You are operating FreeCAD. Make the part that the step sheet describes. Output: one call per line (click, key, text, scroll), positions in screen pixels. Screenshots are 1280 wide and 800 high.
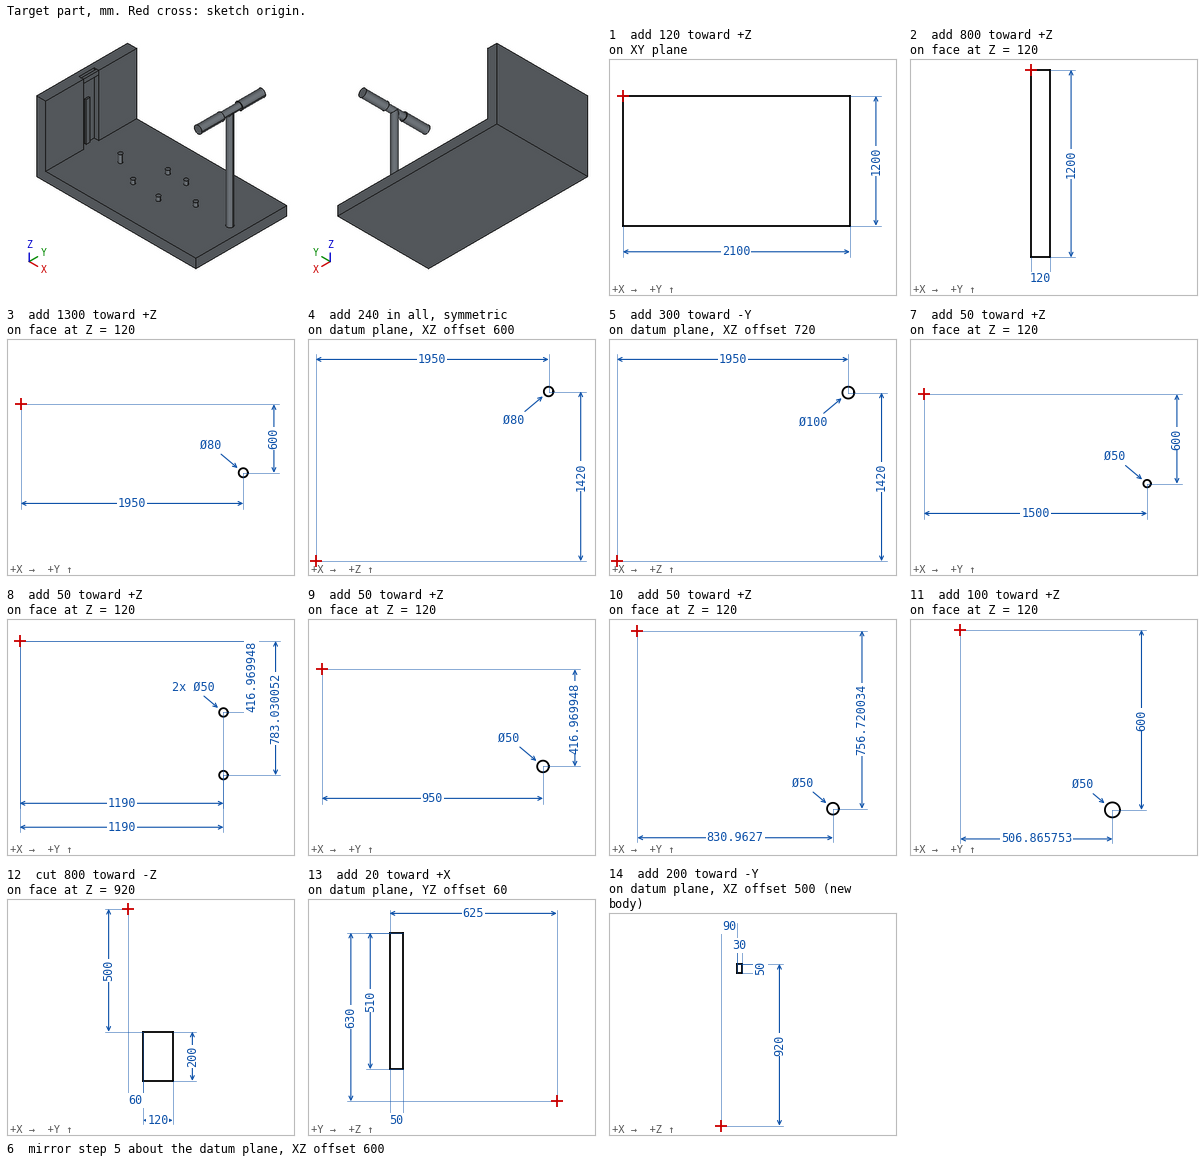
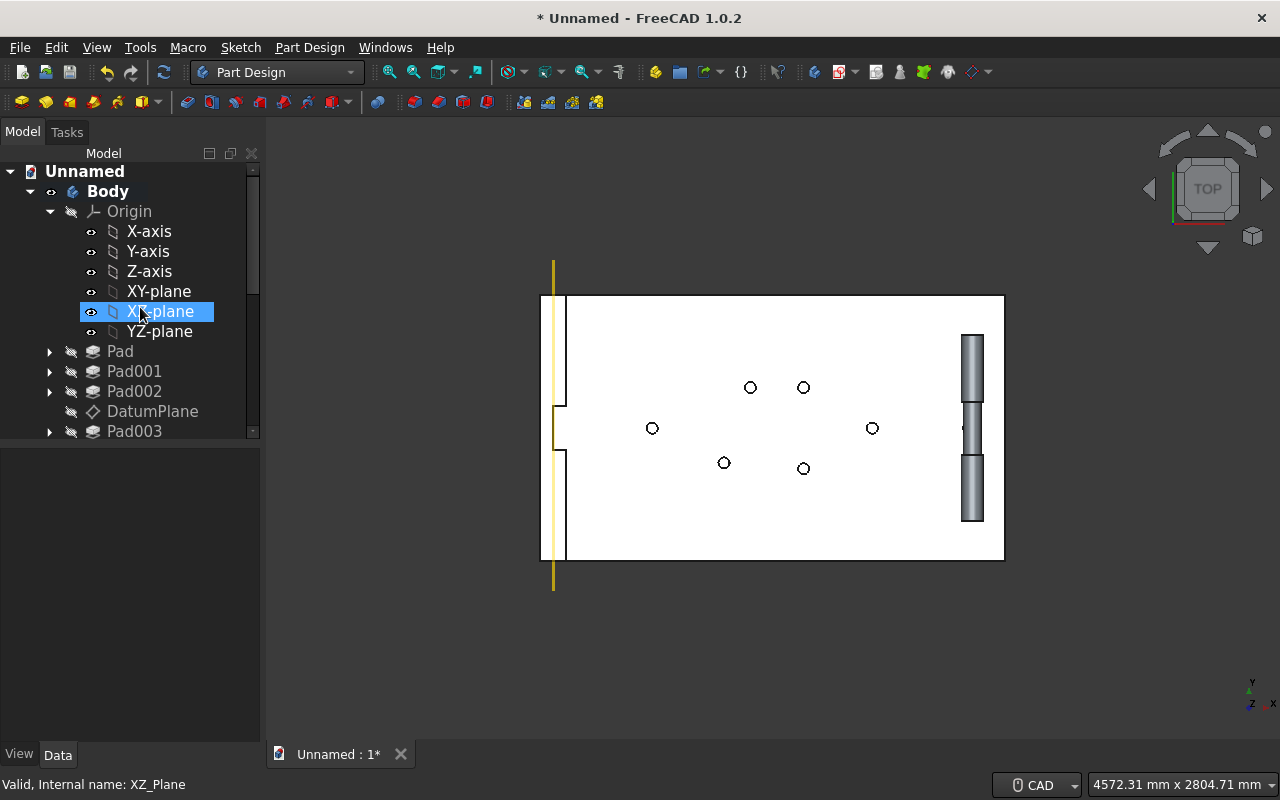
scroll(100, 307, down, 6)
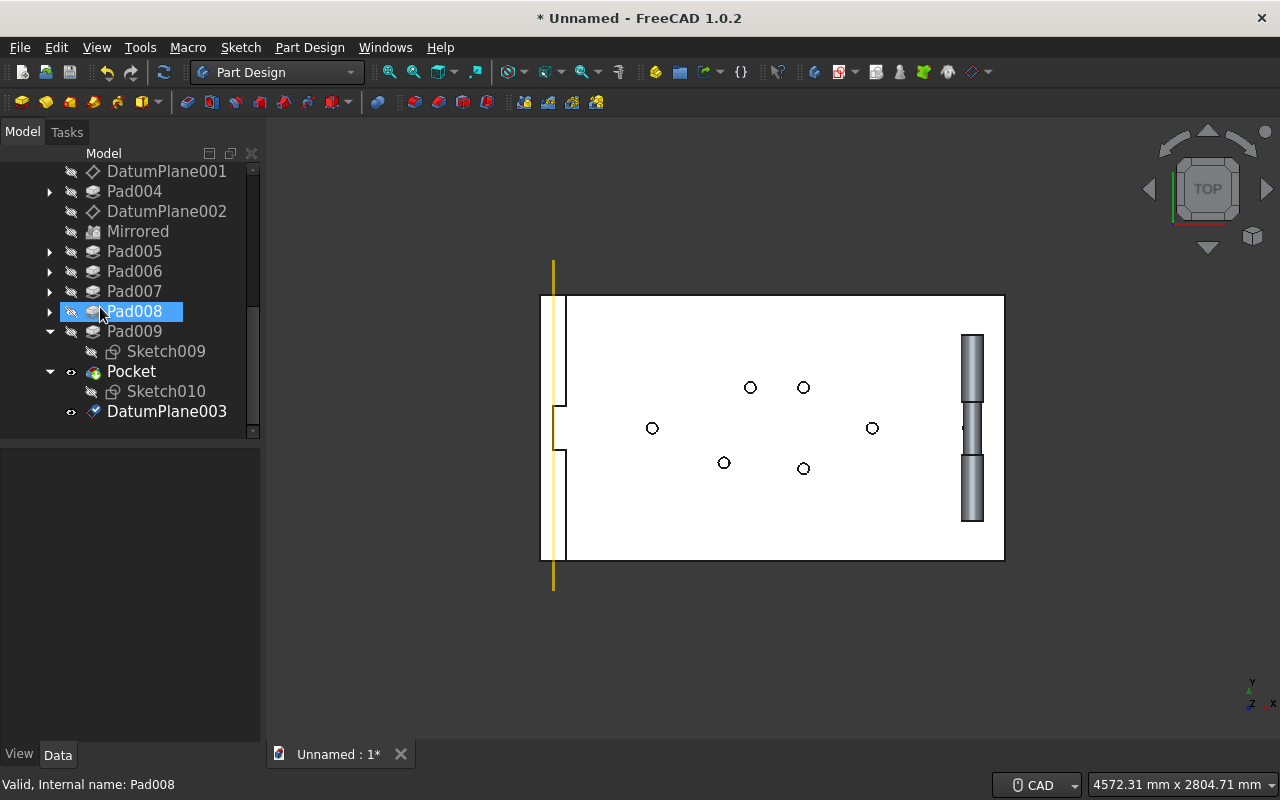
click(116, 412)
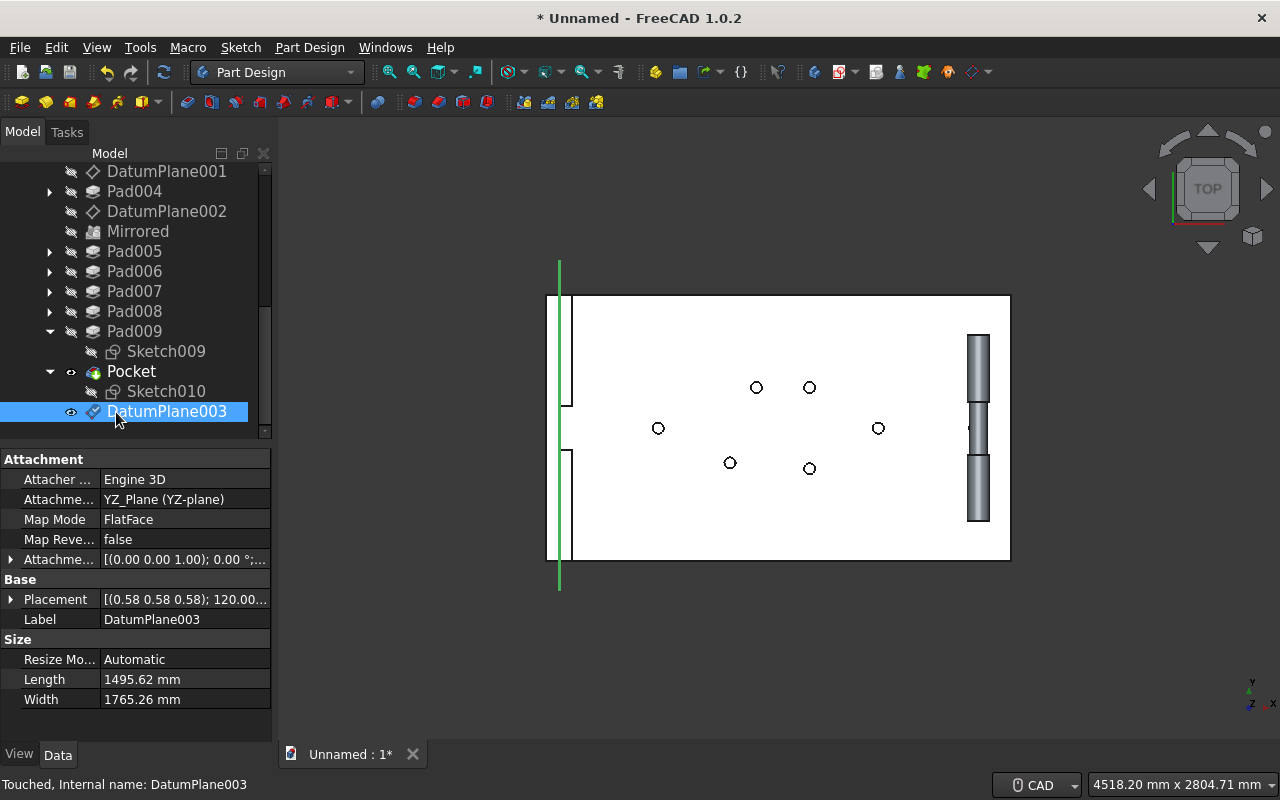
click(840, 72)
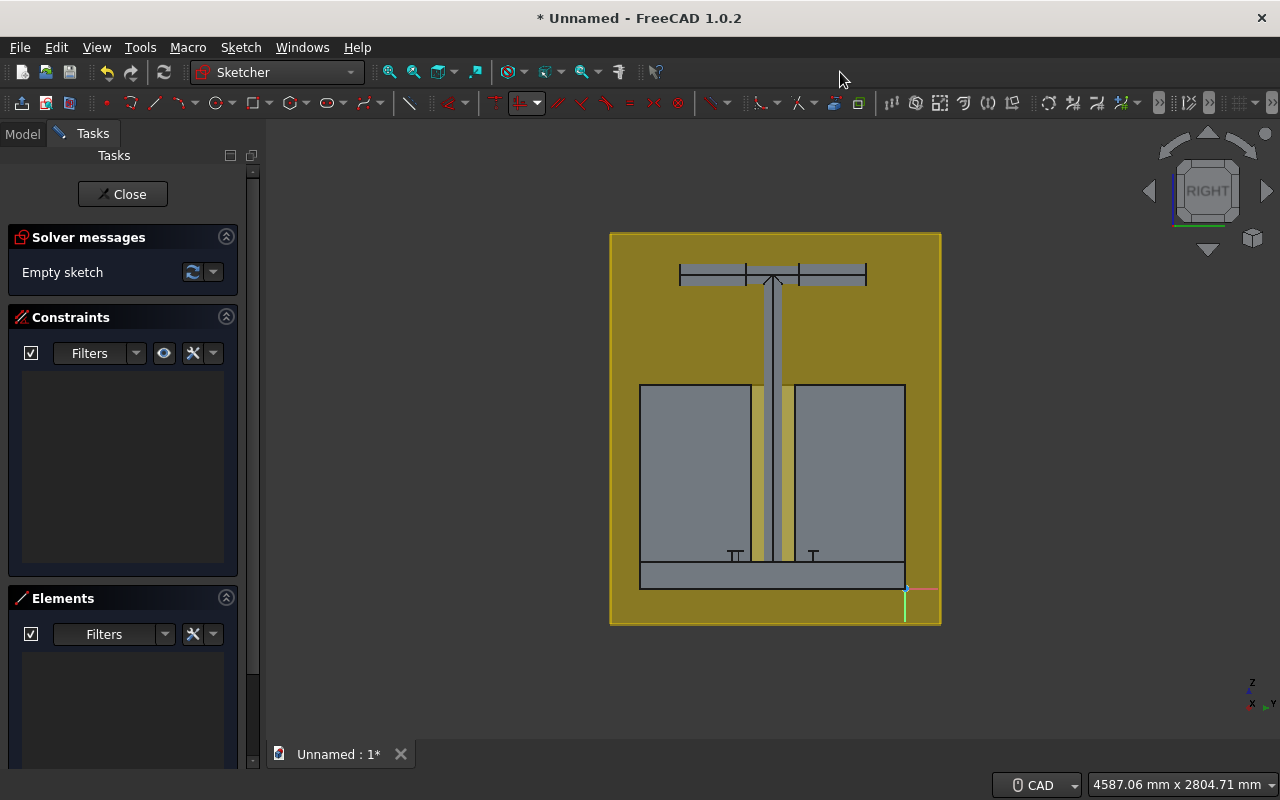
click(70, 104)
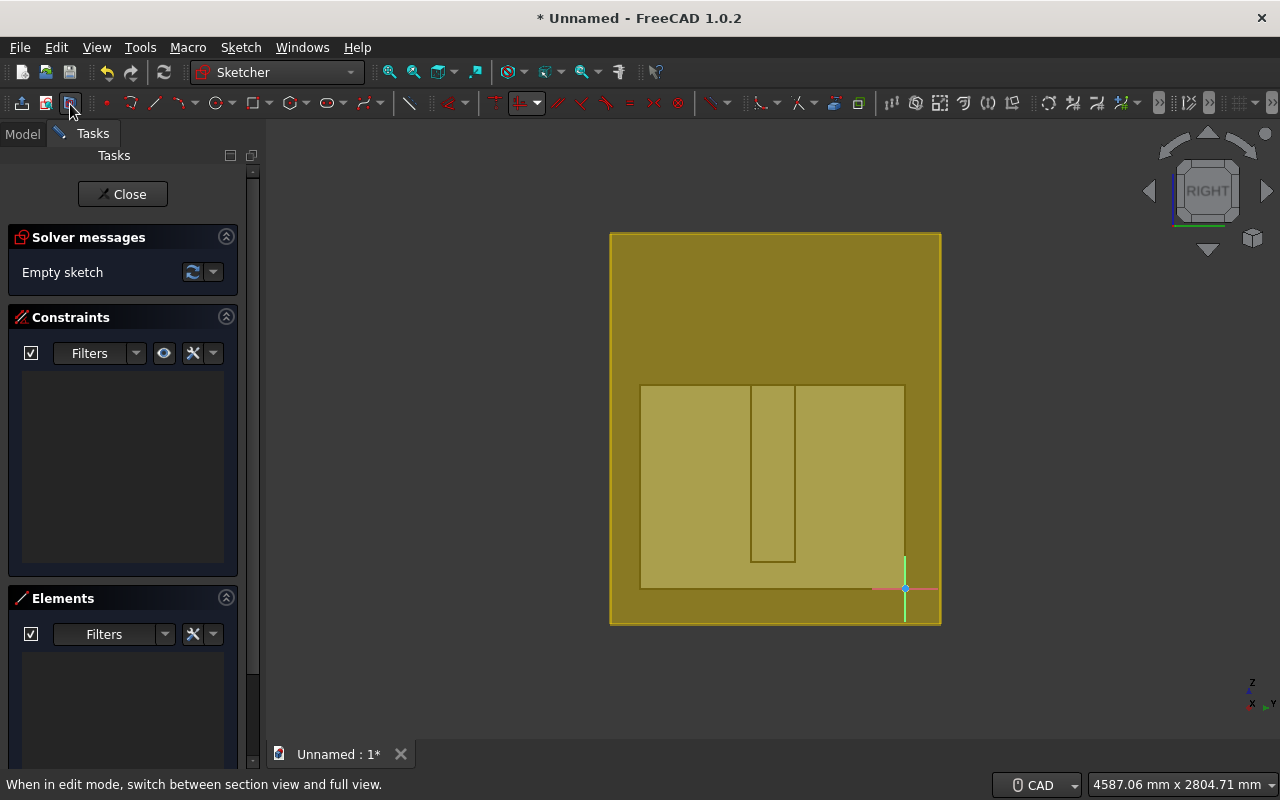
scroll(913, 571, up, 5)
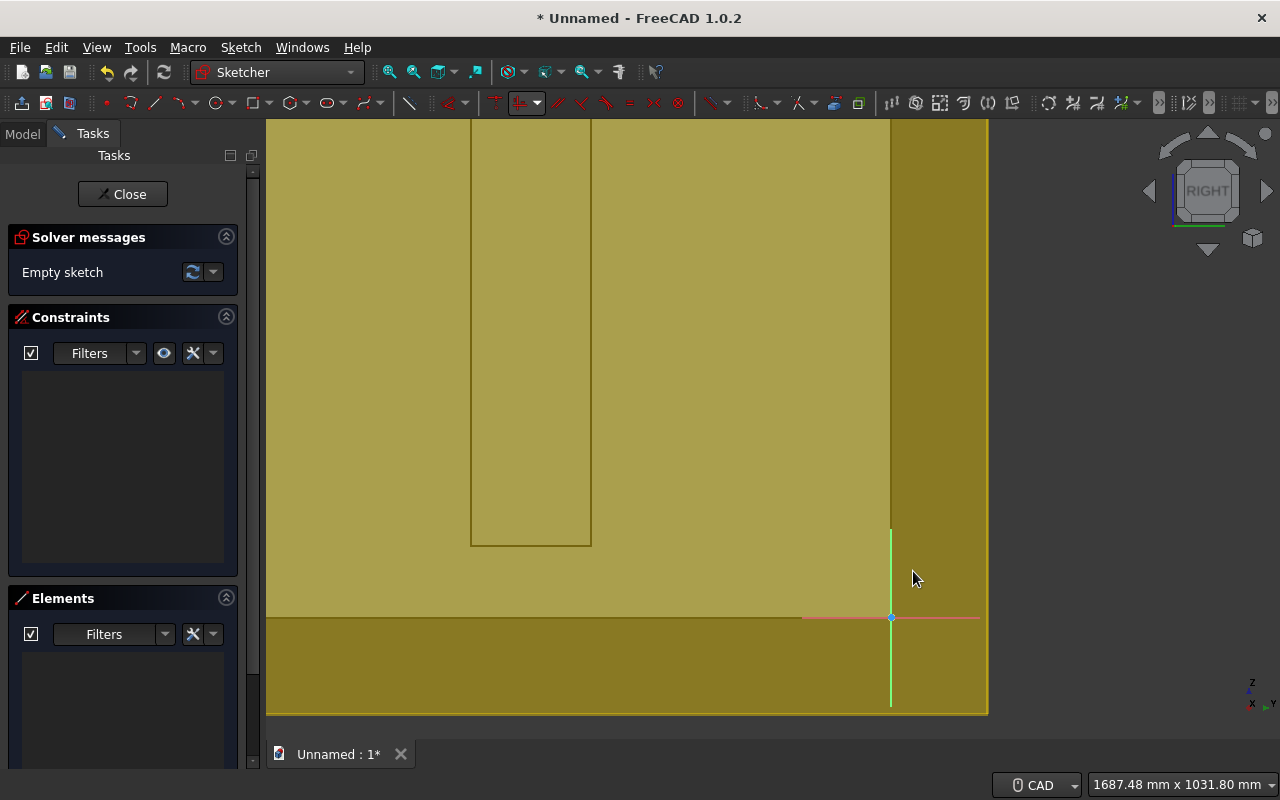
click(254, 104)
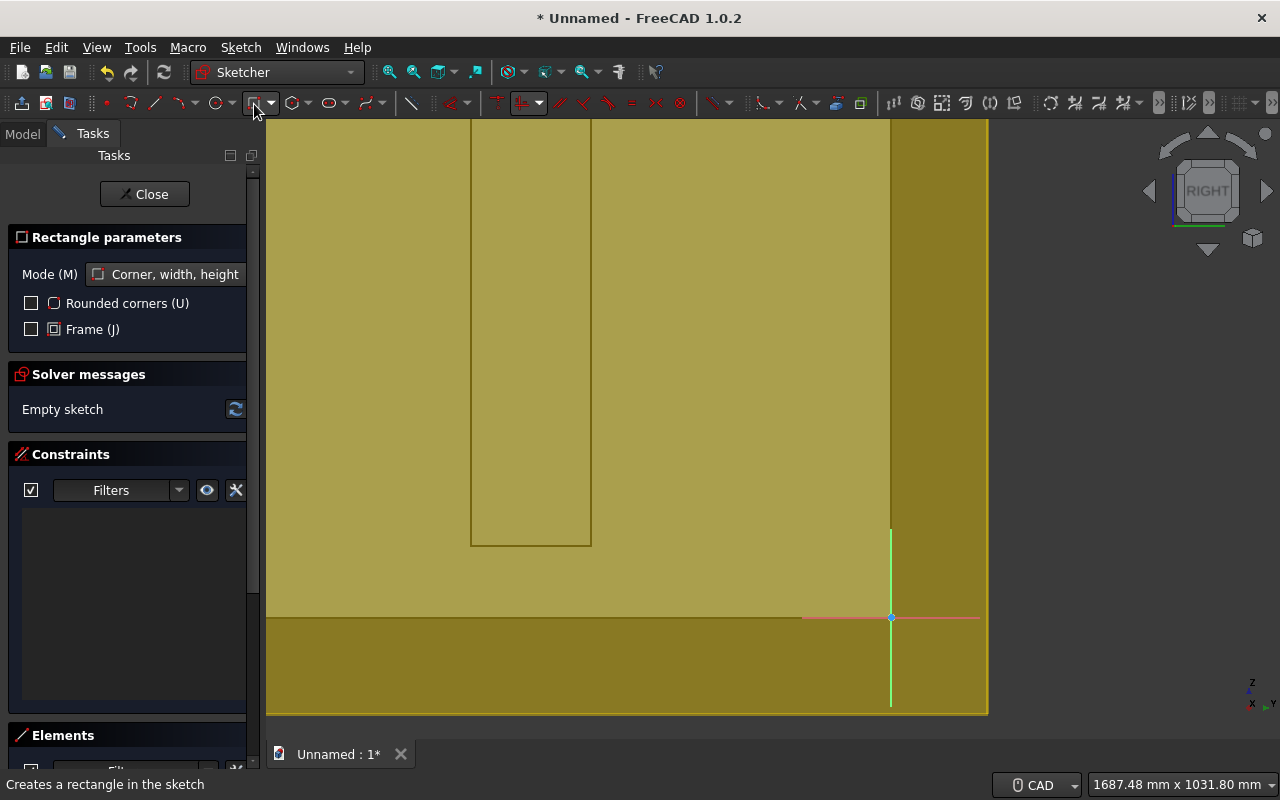
click(516, 239)
move(546, 546)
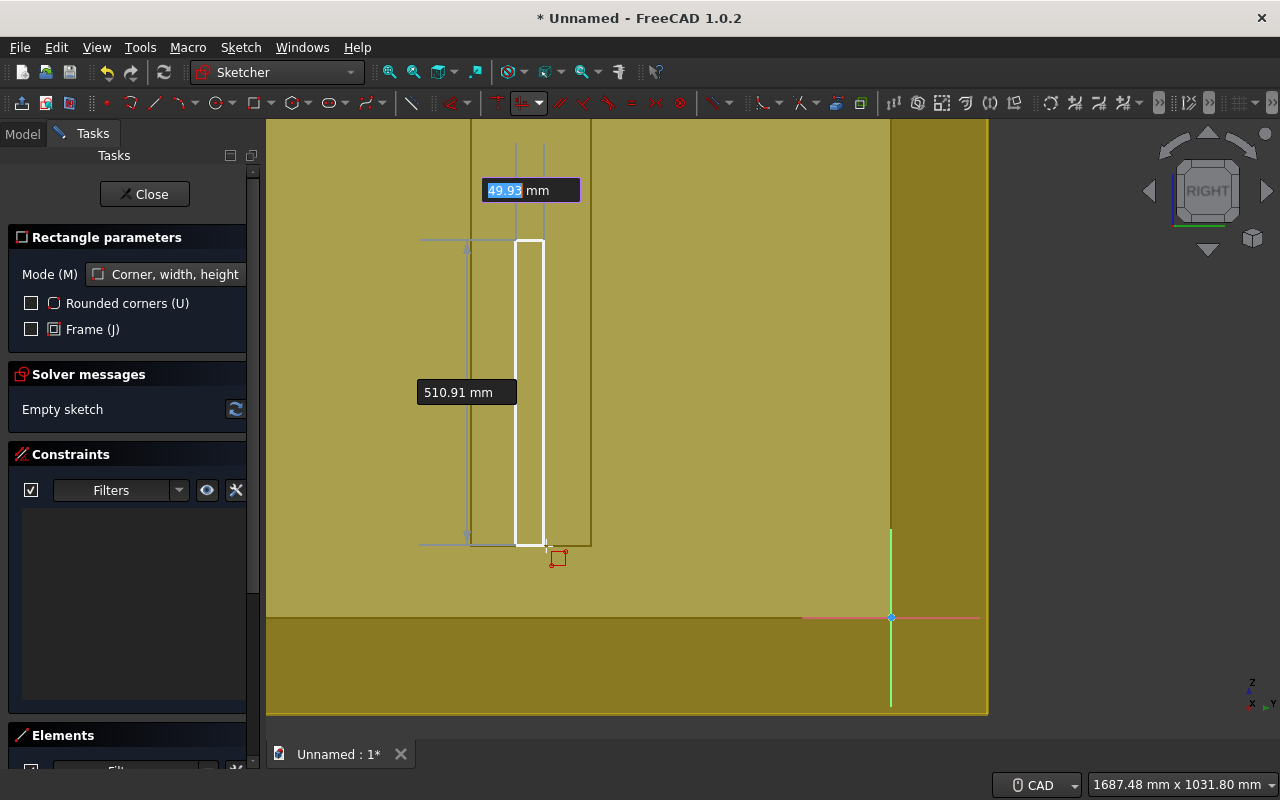
text(50)
key(Tab)
text(510)
key(Return)
key(Escape)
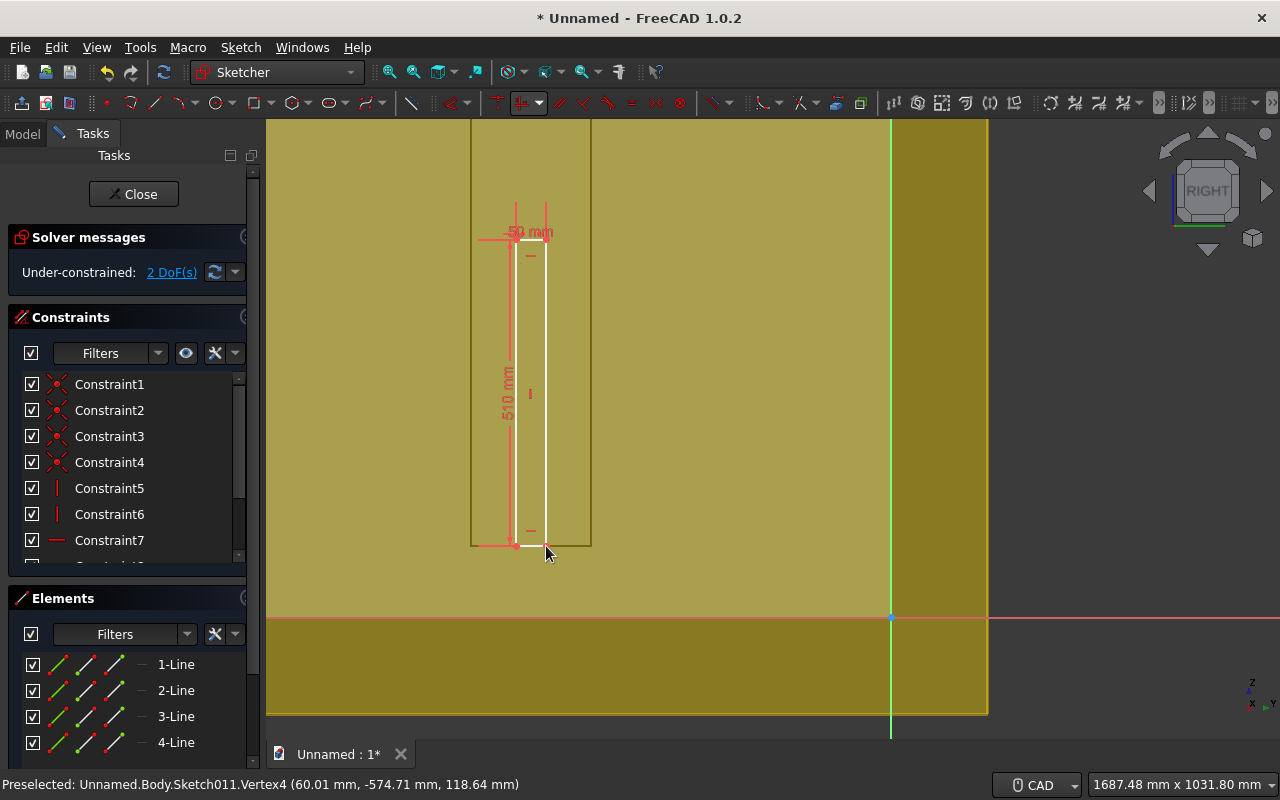
click(450, 104)